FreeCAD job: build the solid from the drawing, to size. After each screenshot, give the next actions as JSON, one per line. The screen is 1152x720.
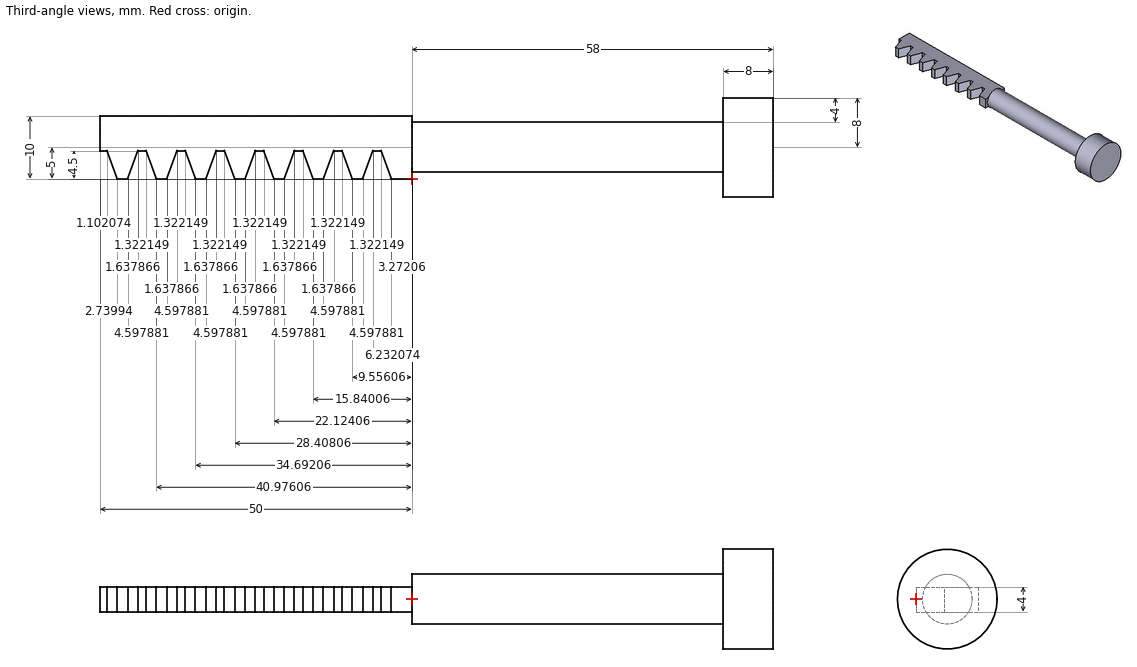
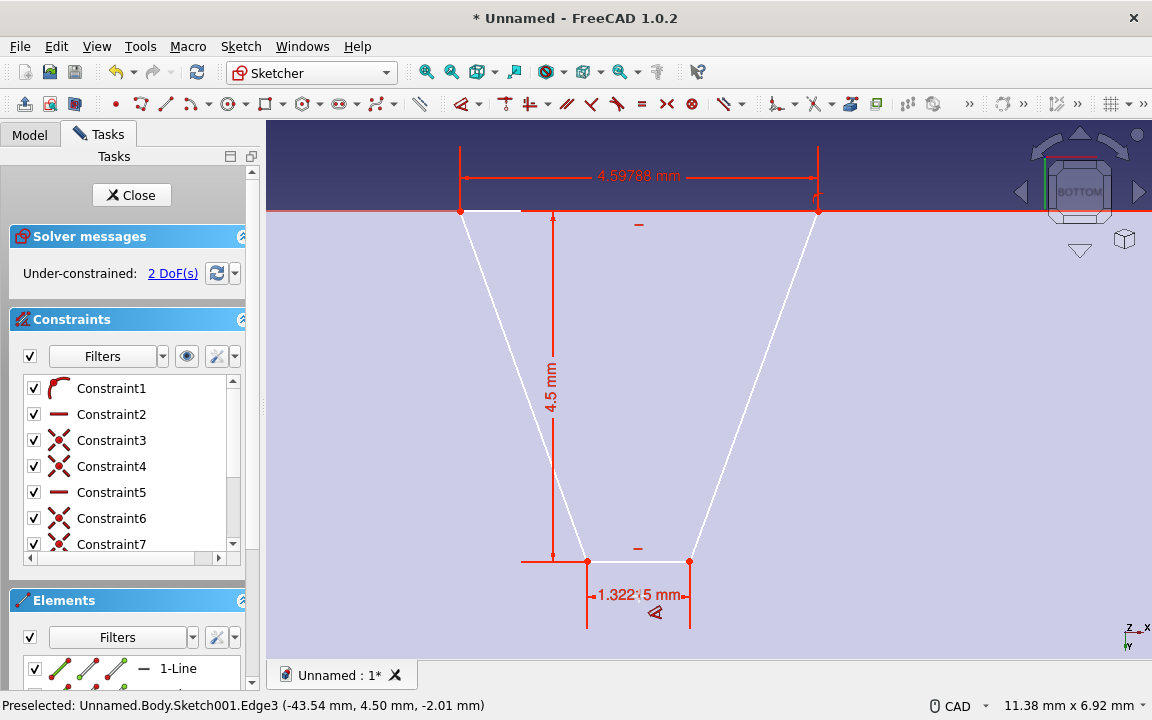
{"action": "left_click", "coordinate": [818, 211]}
{"action": "left_click", "coordinate": [903, 177]}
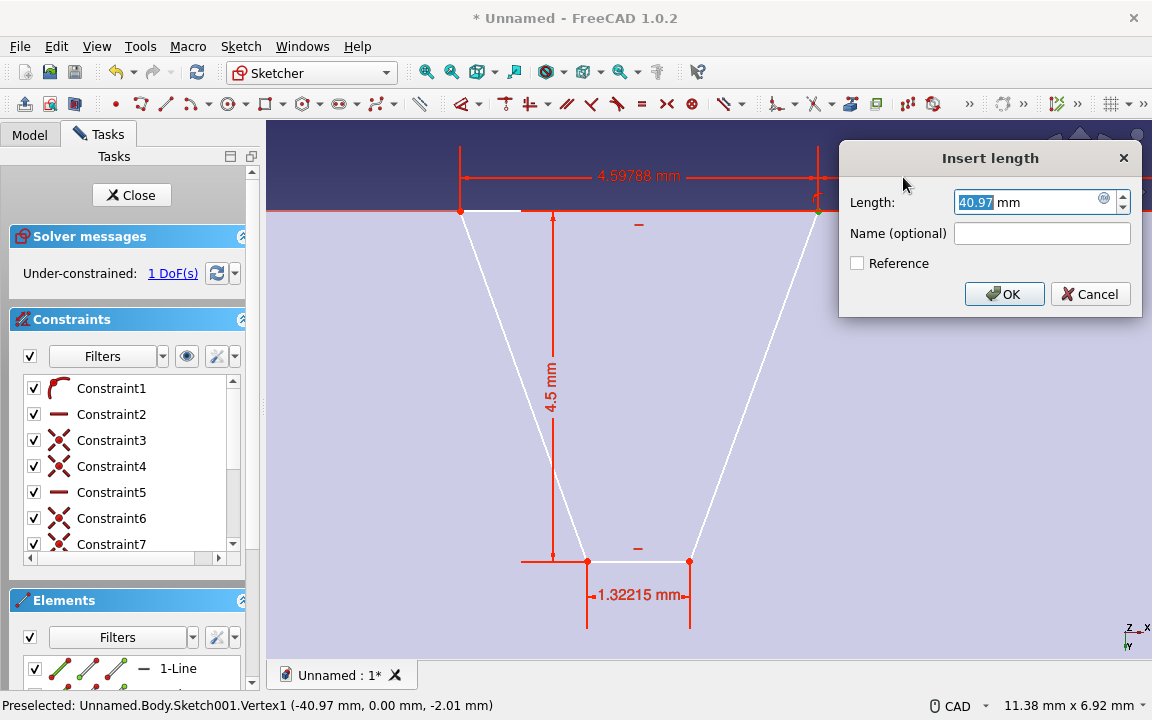
{"action": "type", "text": "40.97606"}
{"action": "key", "text": "Return"}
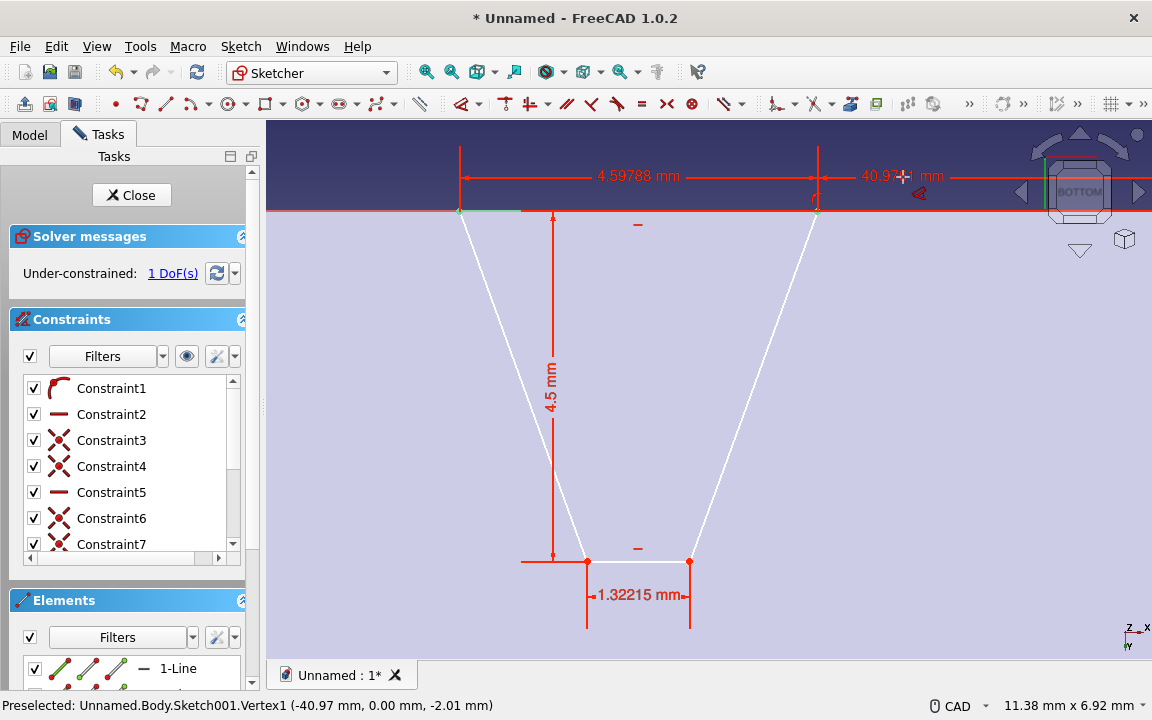
{"action": "left_click", "coordinate": [498, 317]}
{"action": "left_click", "coordinate": [523, 596]}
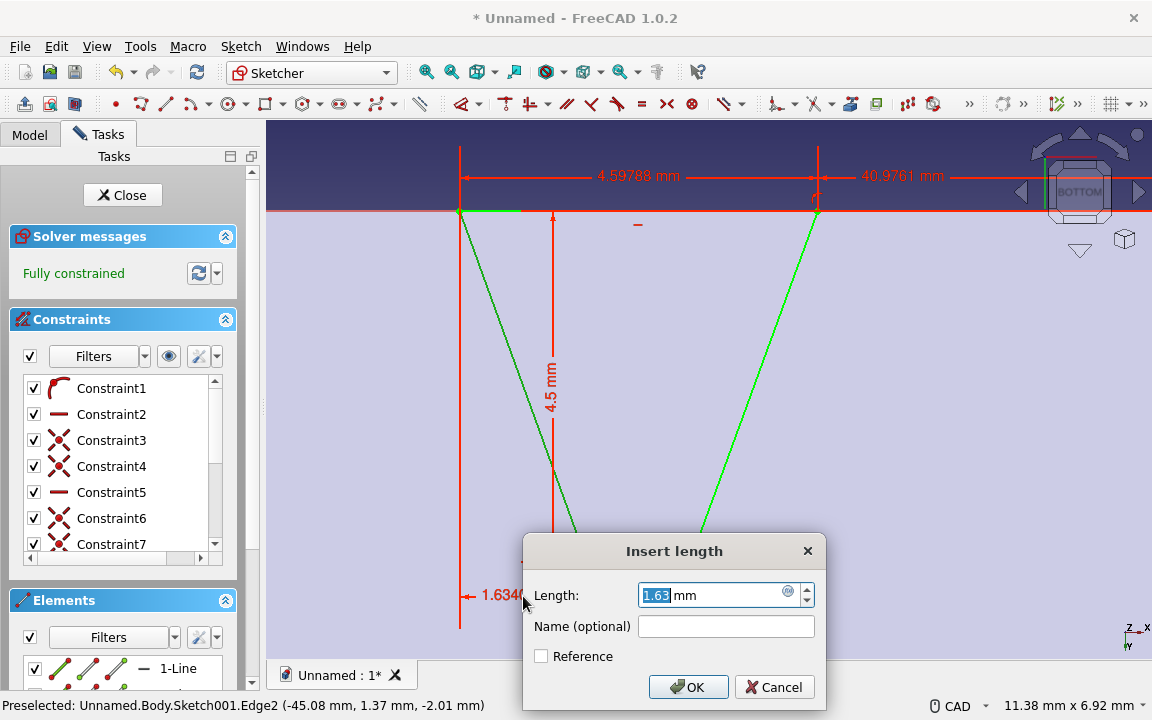
{"action": "type", "text": "1.637866"}
{"action": "key", "text": "Return"}
{"action": "key", "text": "Escape"}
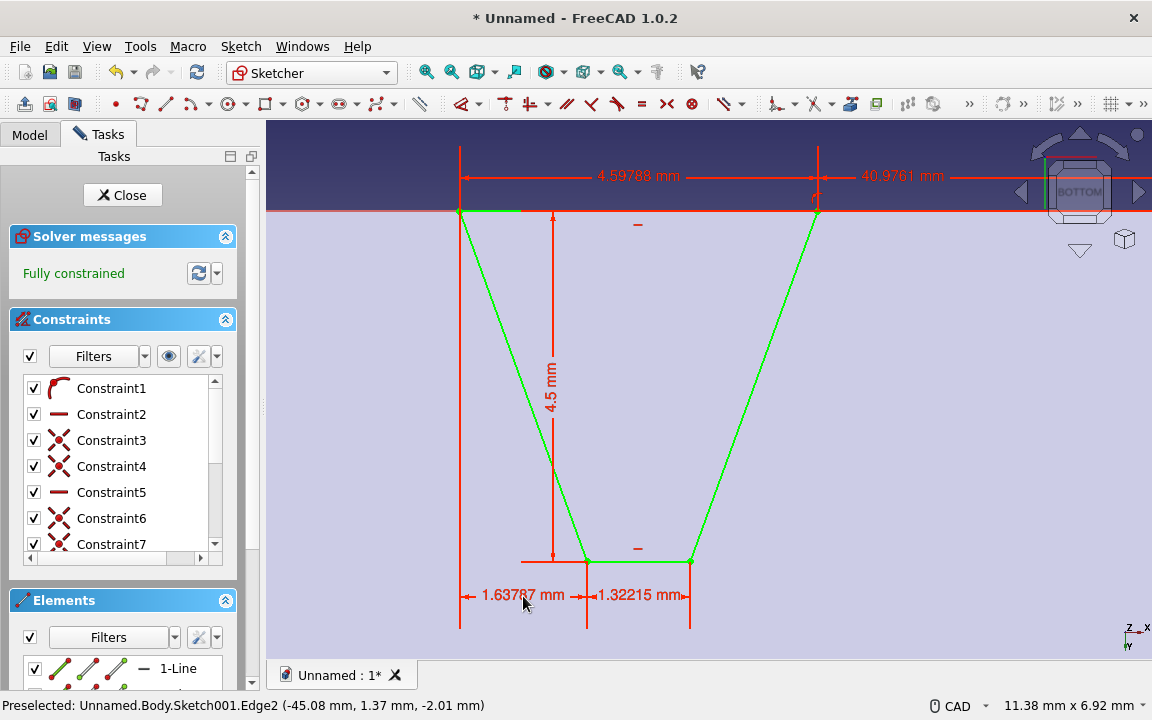
{"action": "left_click", "coordinate": [123, 195]}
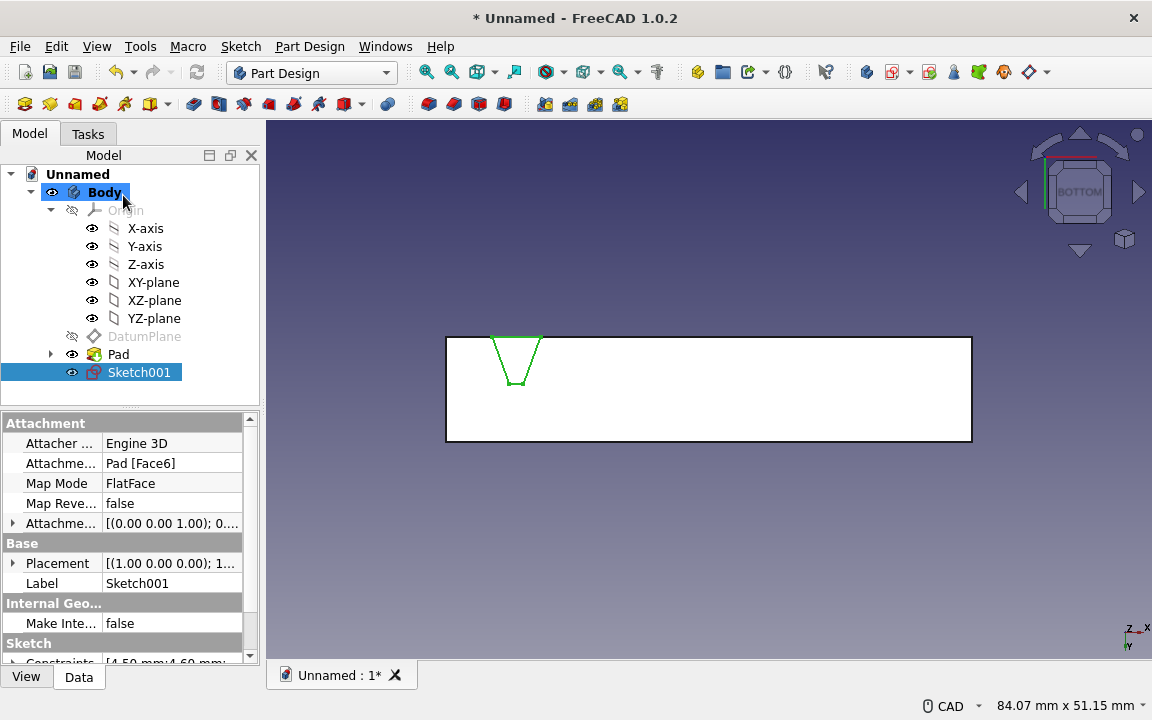
{"action": "left_click", "coordinate": [194, 104]}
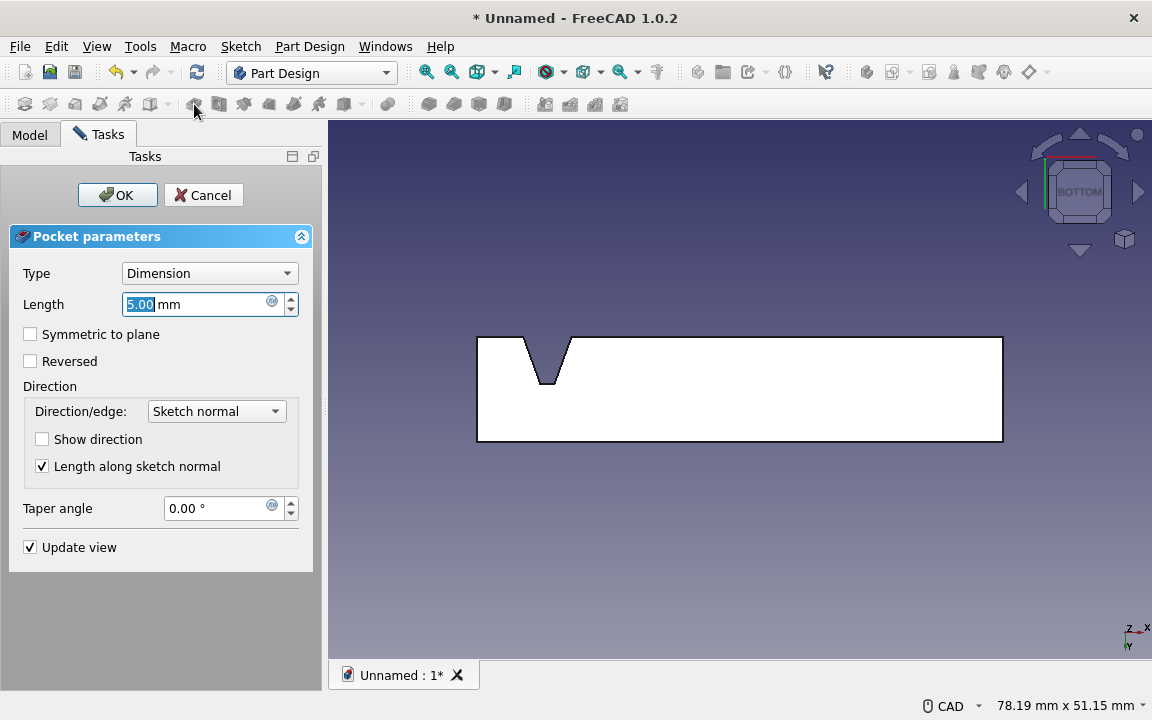
{"action": "left_click", "coordinate": [210, 274]}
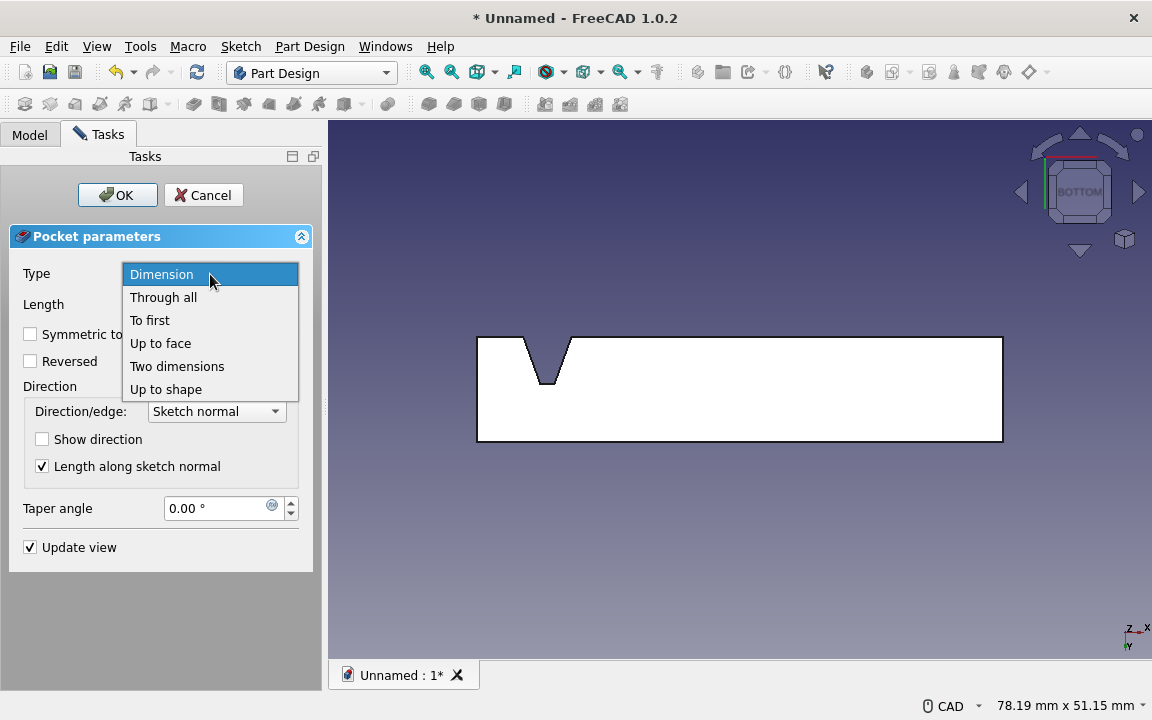
{"action": "left_click", "coordinate": [208, 298]}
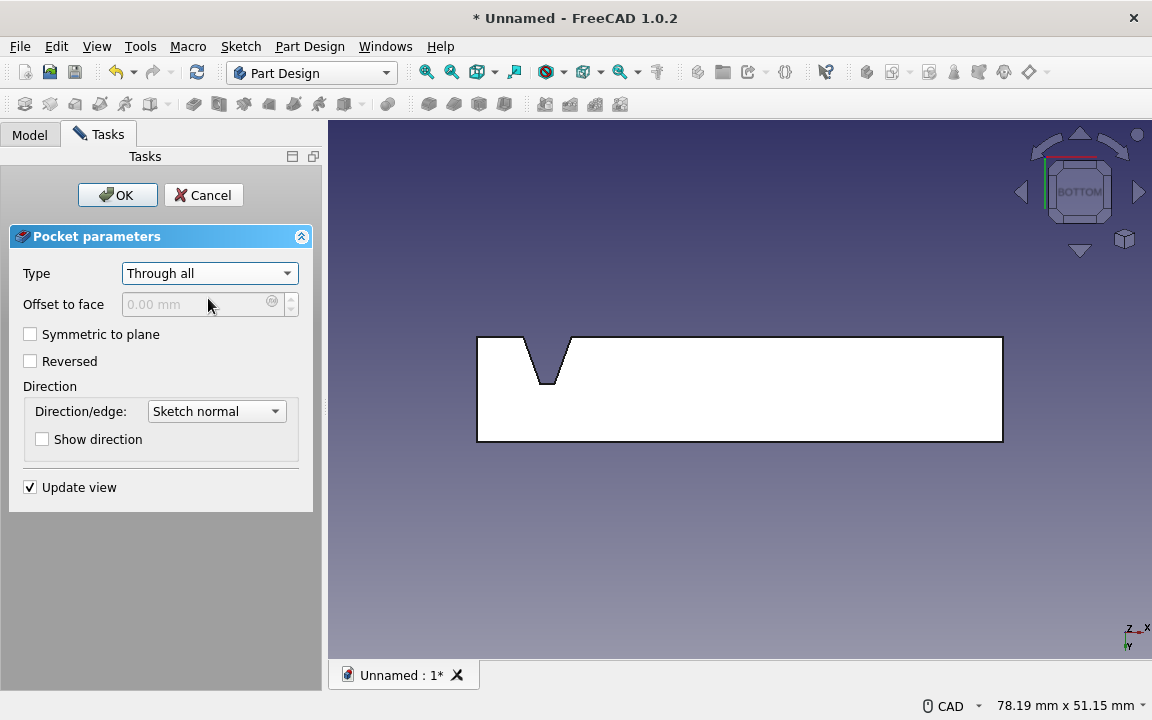
{"action": "left_click", "coordinate": [118, 195]}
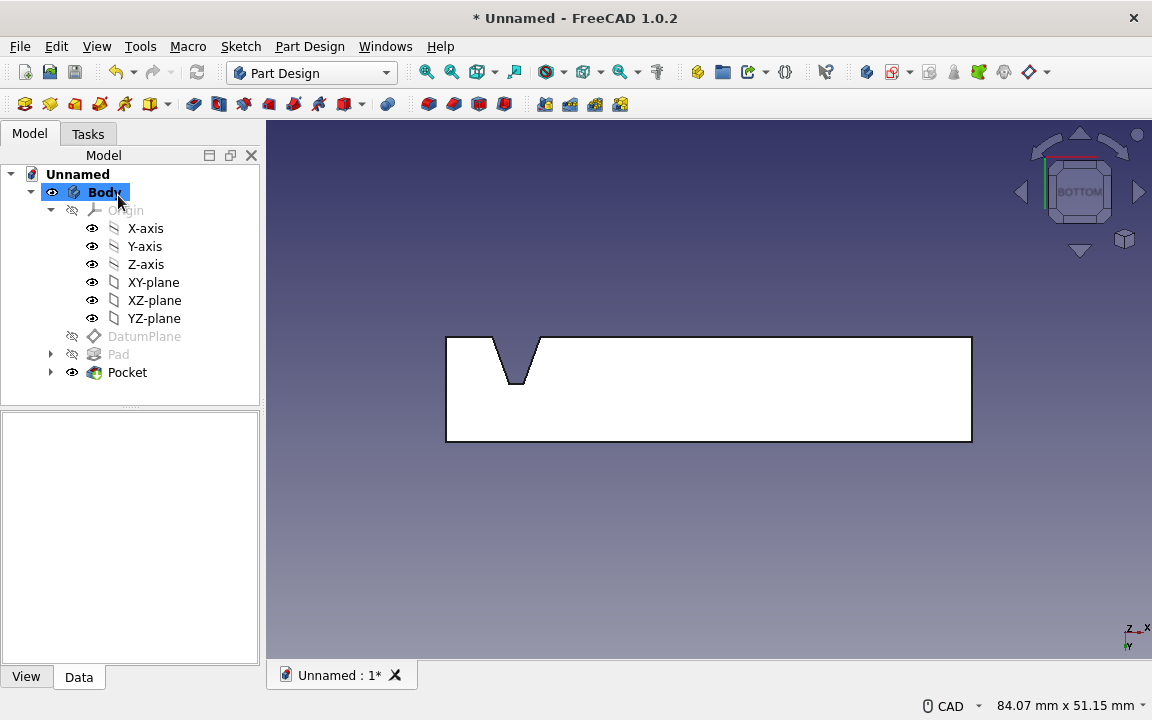
{"action": "left_click", "coordinate": [860, 389]}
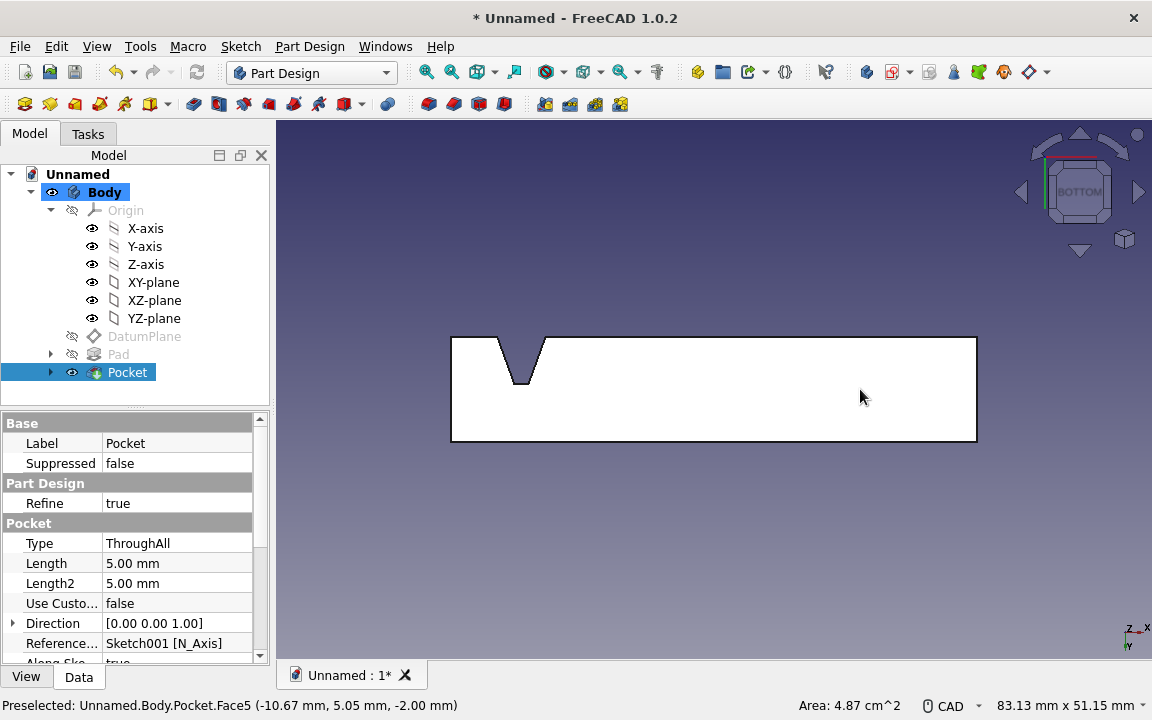
{"action": "left_click", "coordinate": [892, 72]}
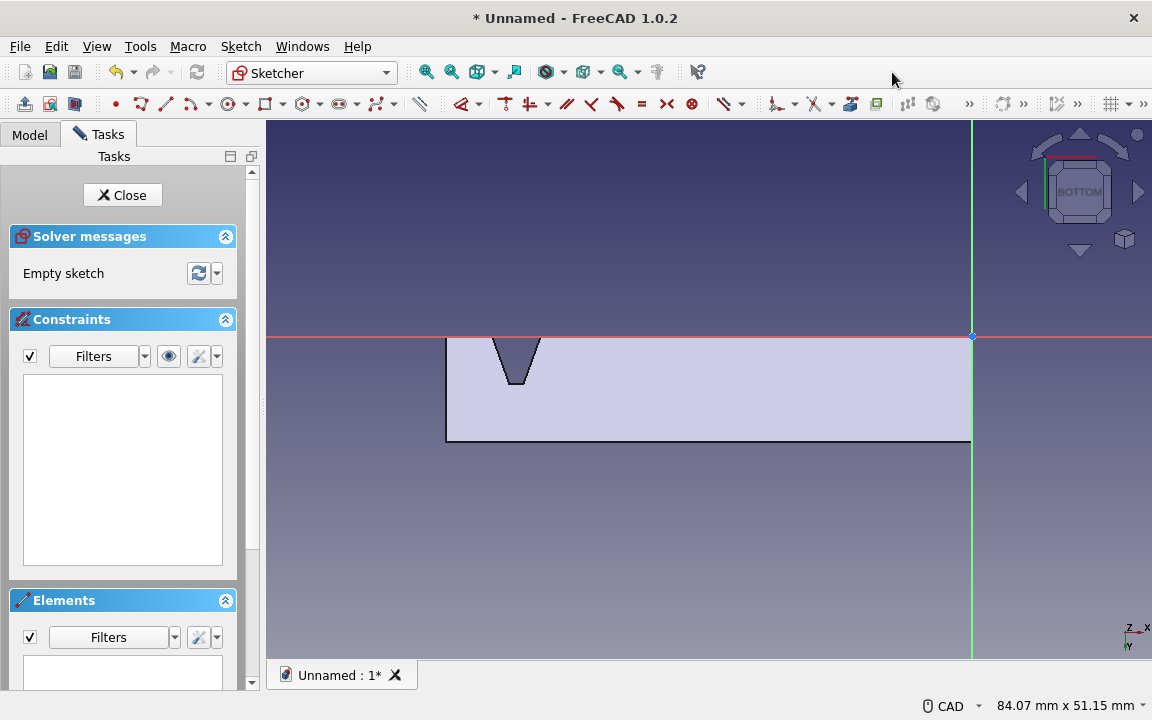
{"action": "scroll", "coordinate": [574, 356], "scroll_direction": "up", "scroll_amount": 10}